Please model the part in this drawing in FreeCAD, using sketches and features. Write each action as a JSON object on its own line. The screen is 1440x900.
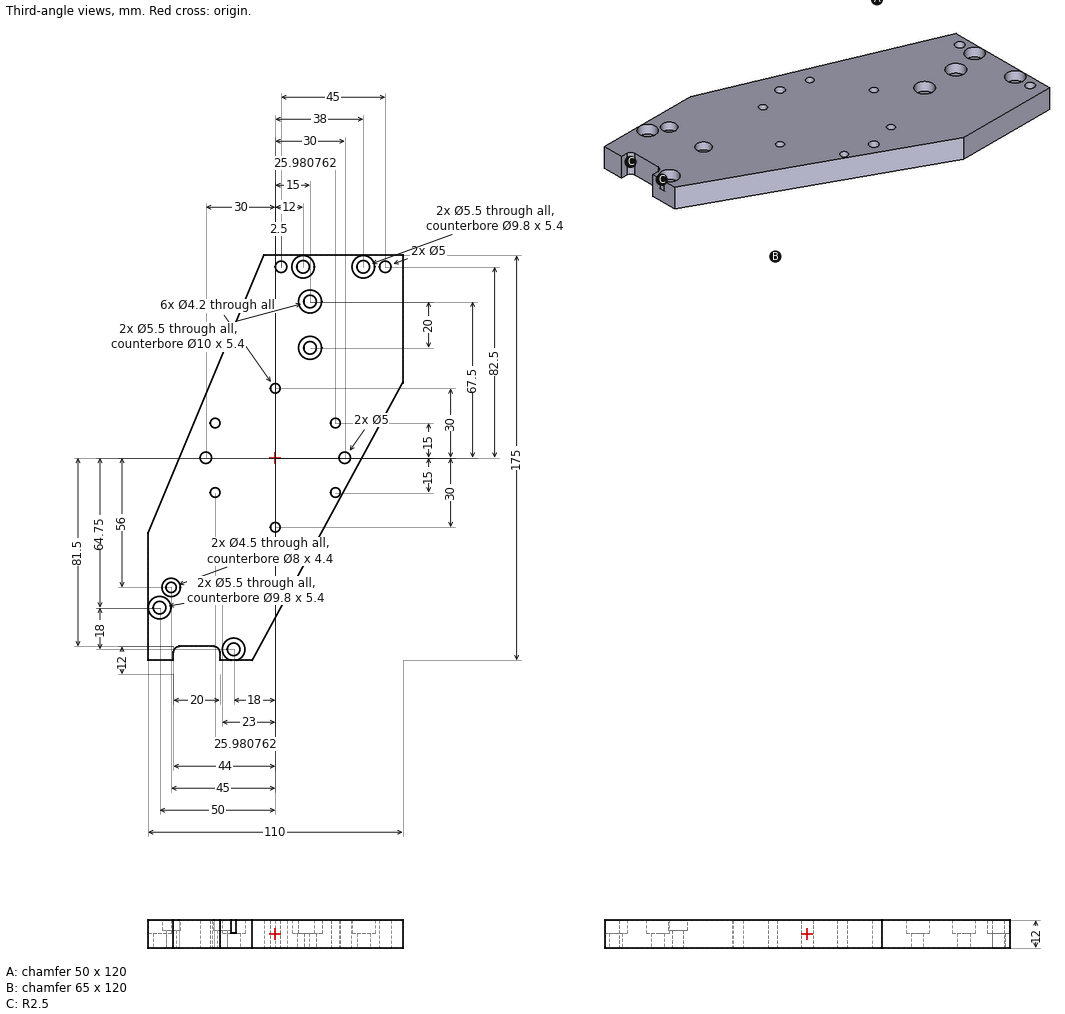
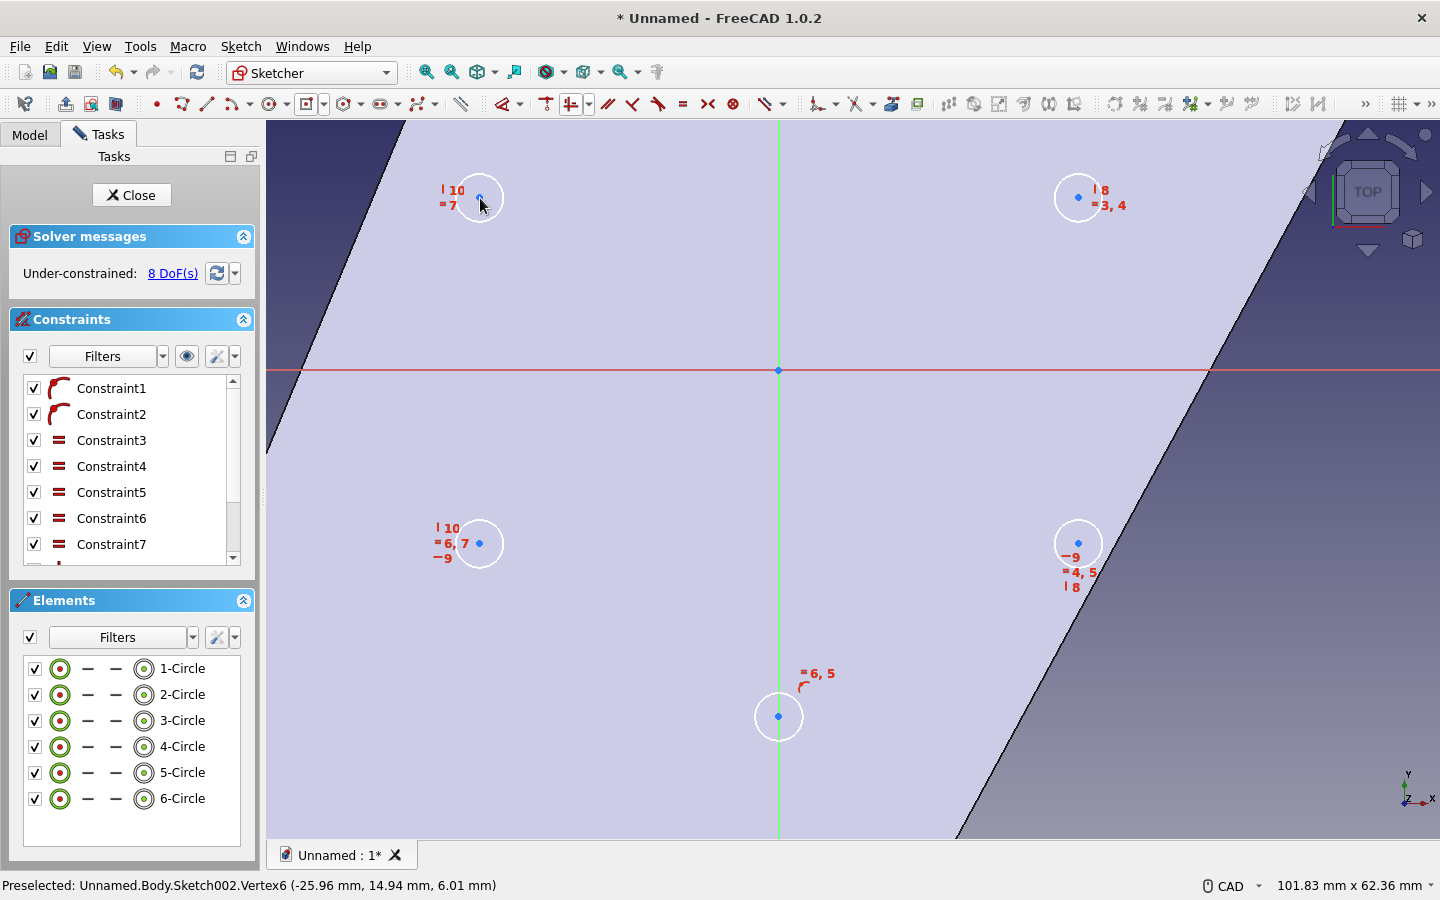
{"action": "left_click", "coordinate": [1079, 198]}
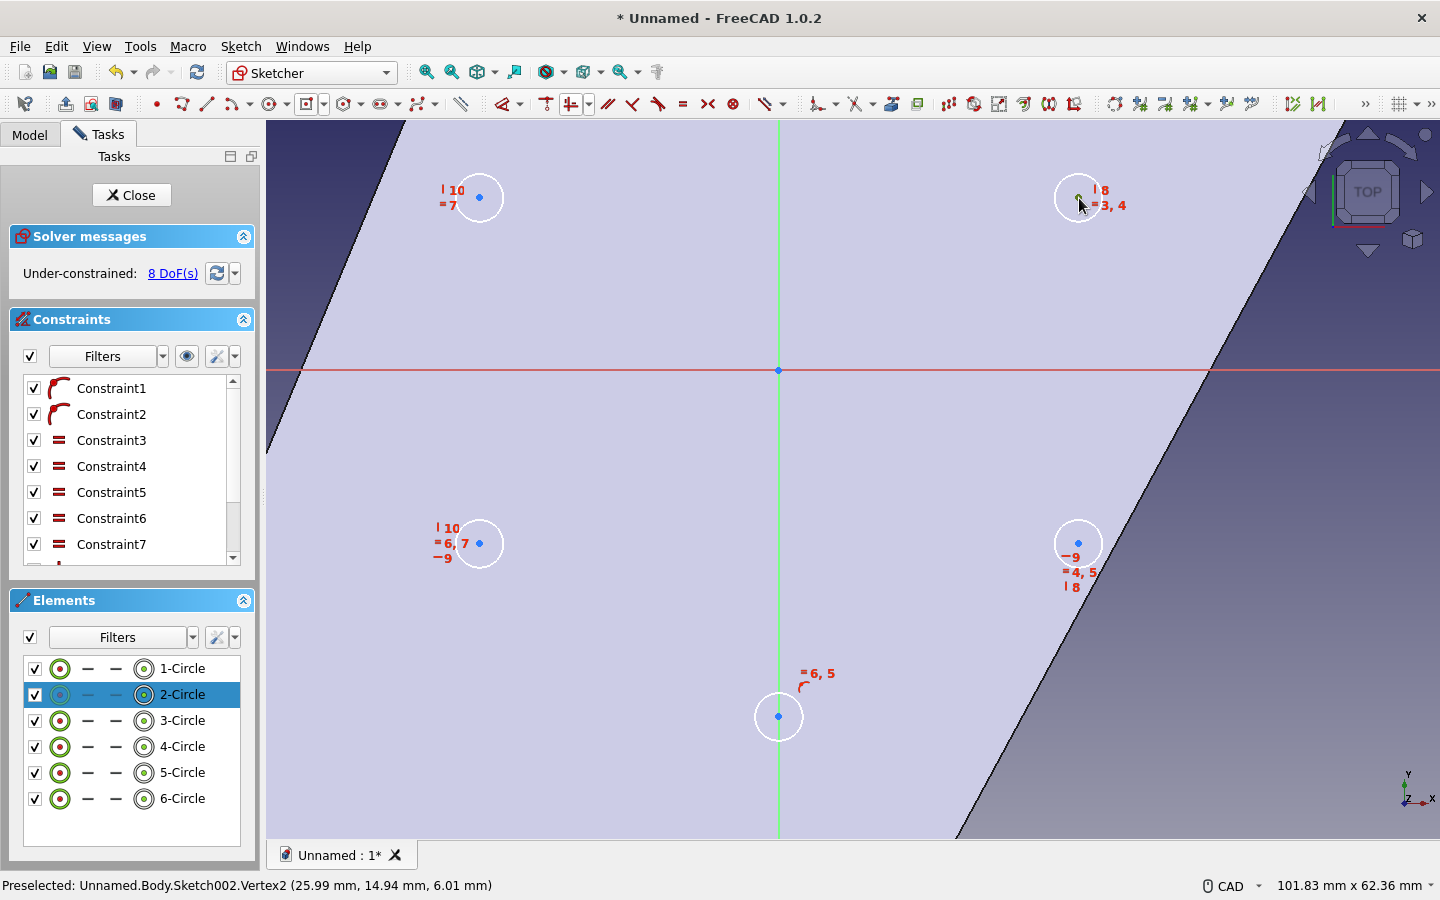
{"action": "left_click", "coordinate": [480, 198]}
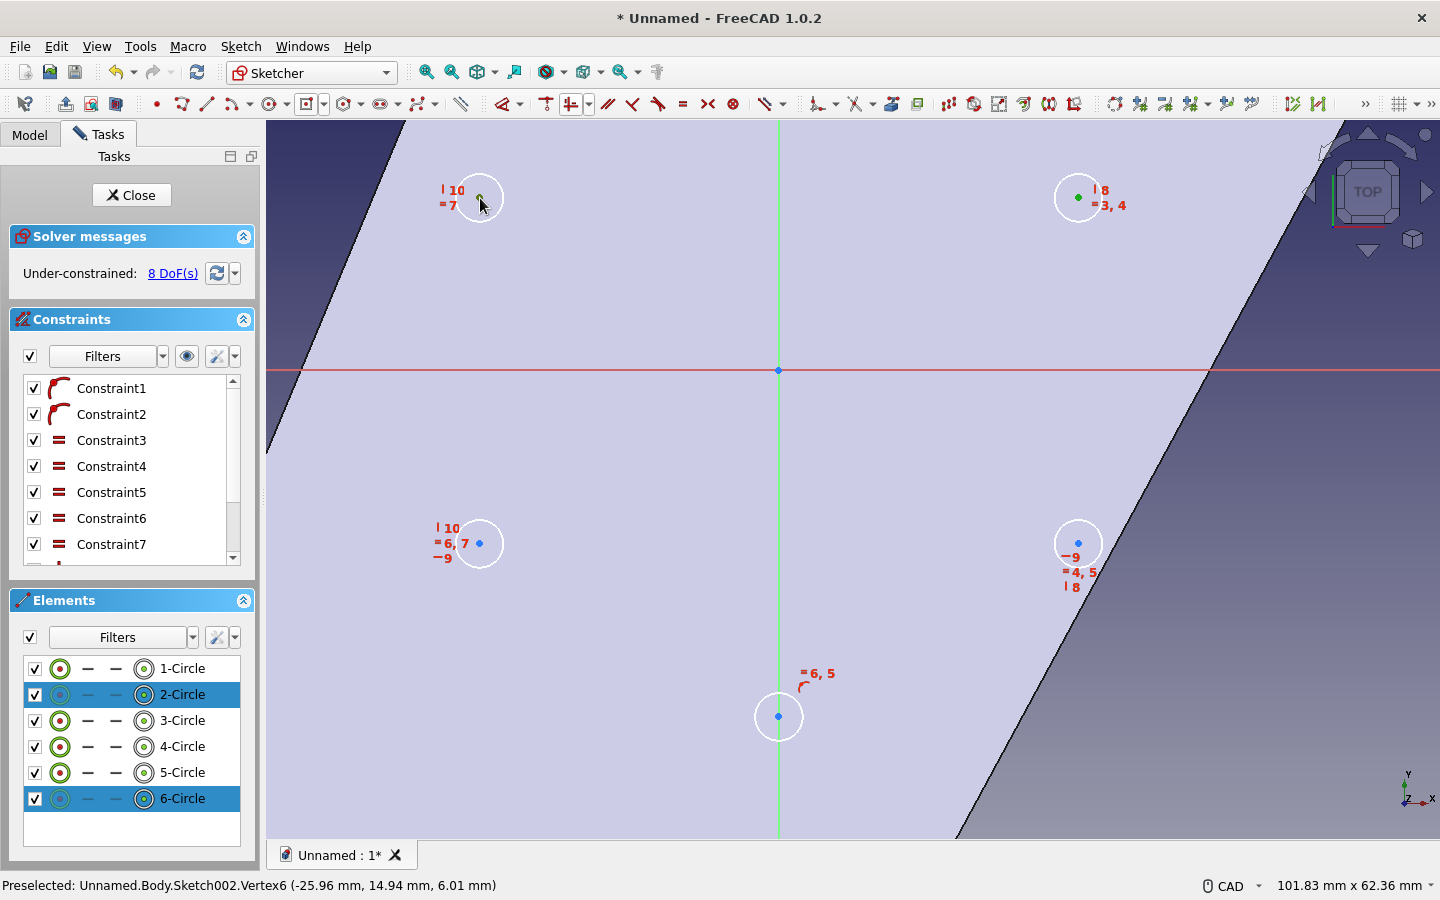
{"action": "key", "text": "h"}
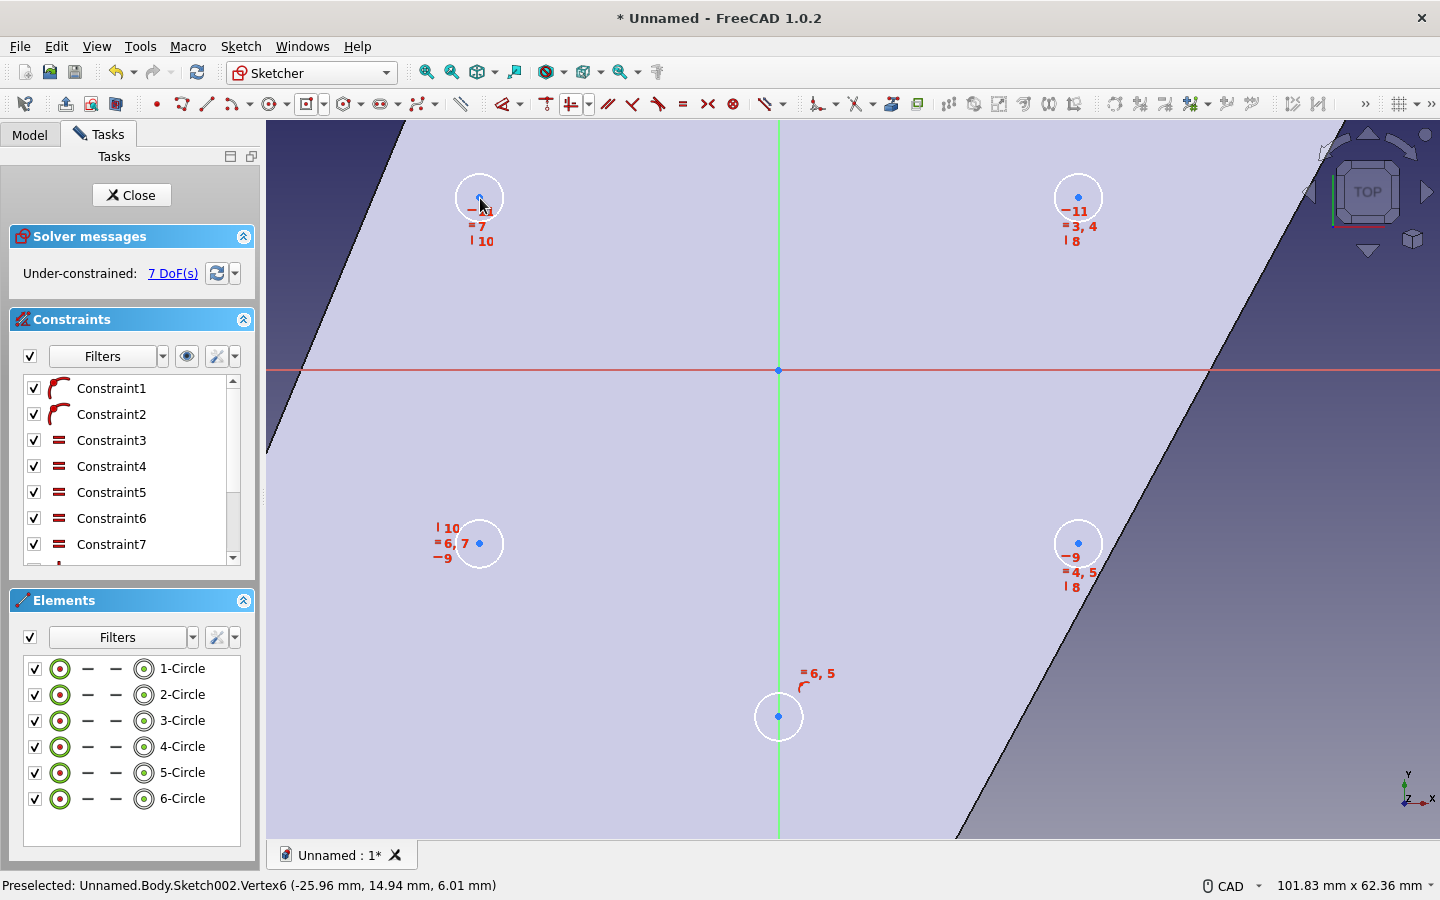
{"action": "scroll", "coordinate": [796, 702], "scroll_direction": "down", "scroll_amount": 2}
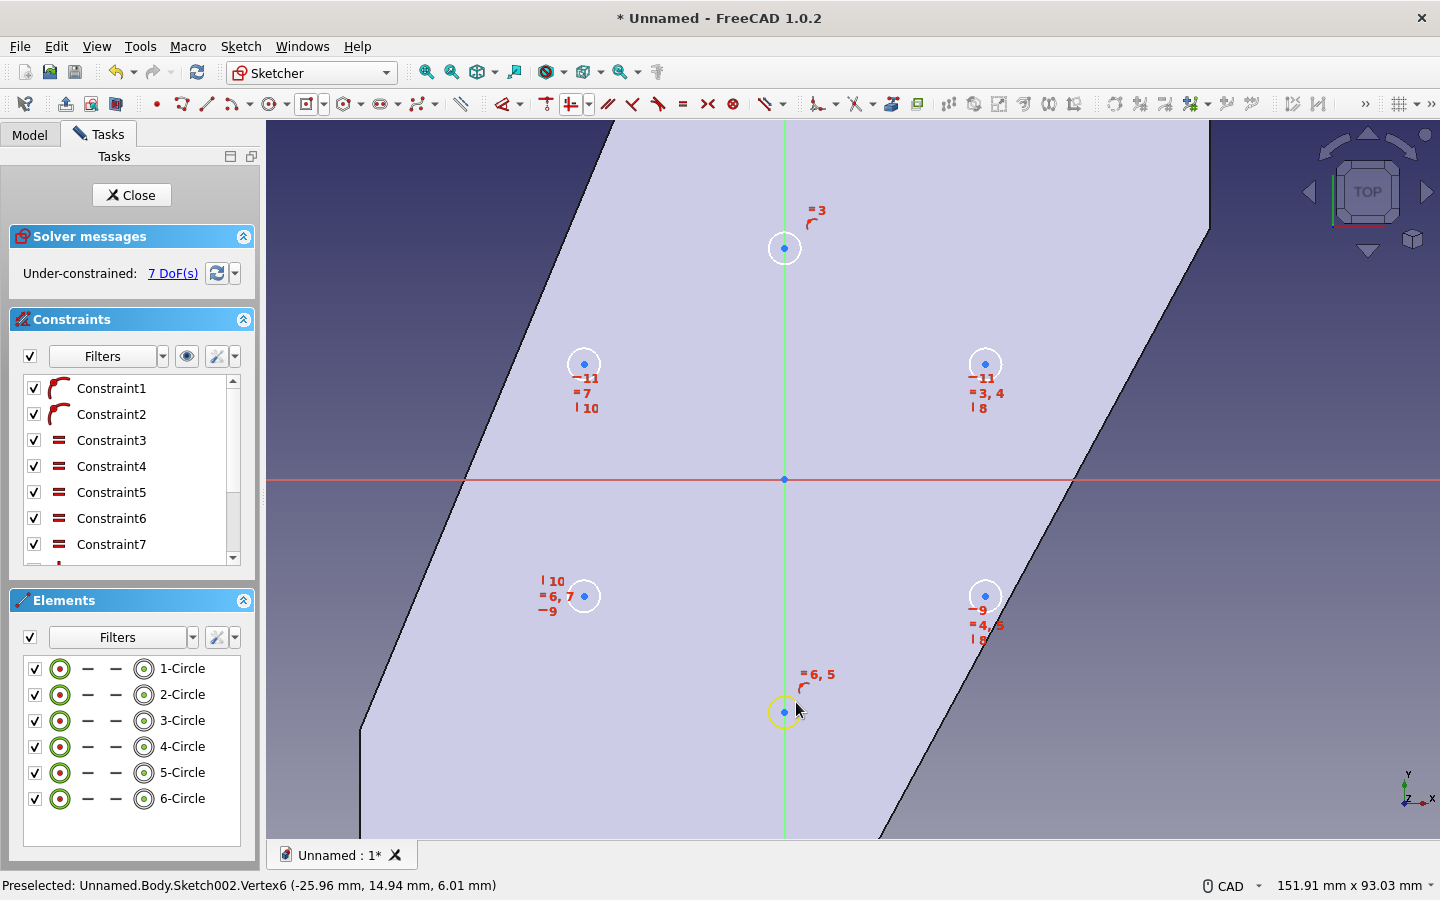
{"action": "scroll", "coordinate": [796, 237], "scroll_direction": "up", "scroll_amount": 2}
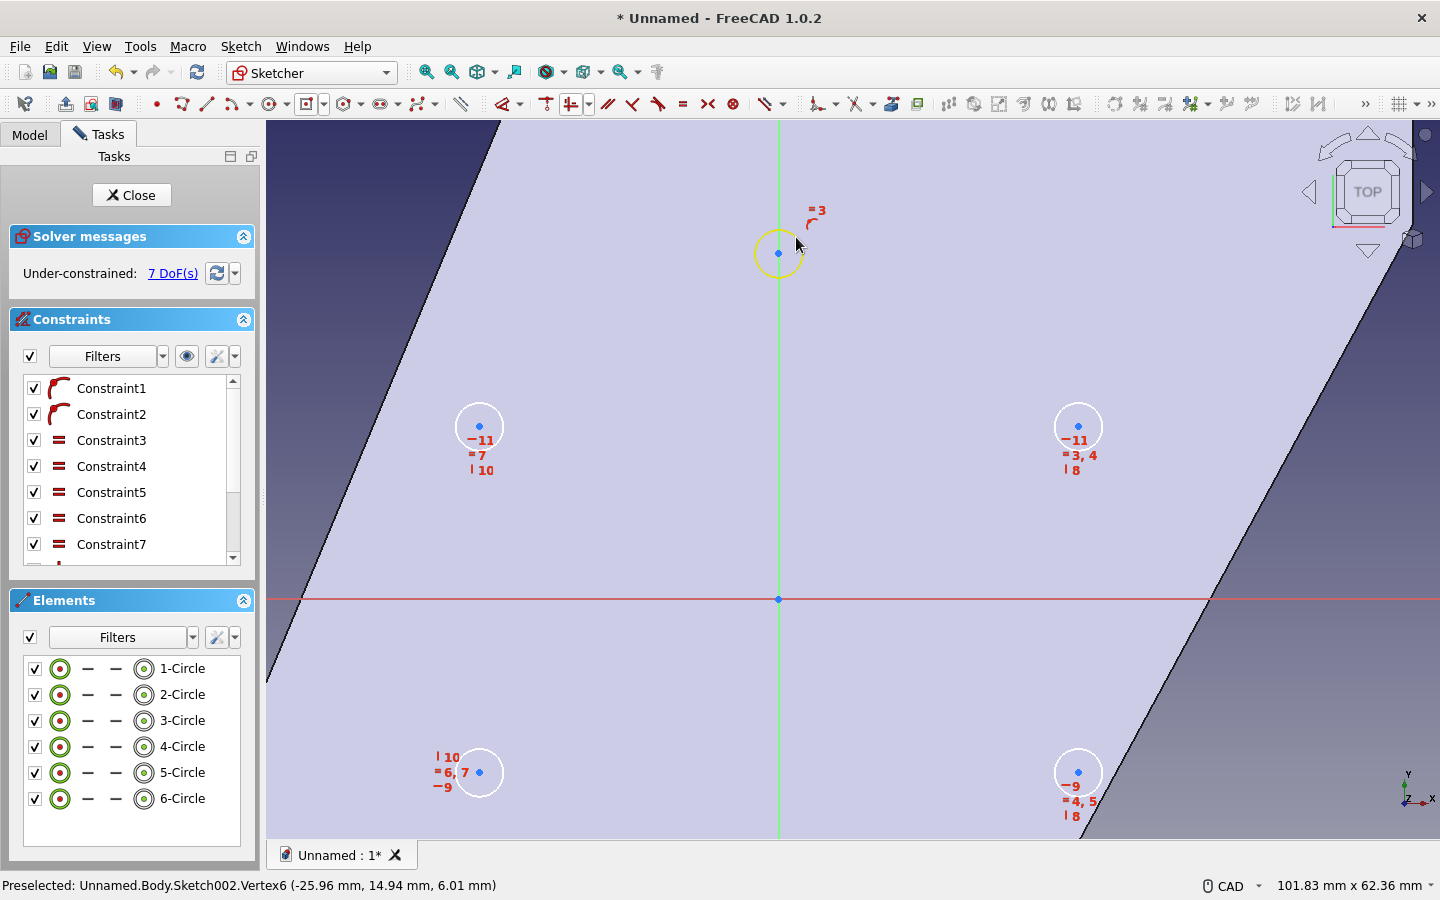
{"action": "left_click", "coordinate": [796, 237]}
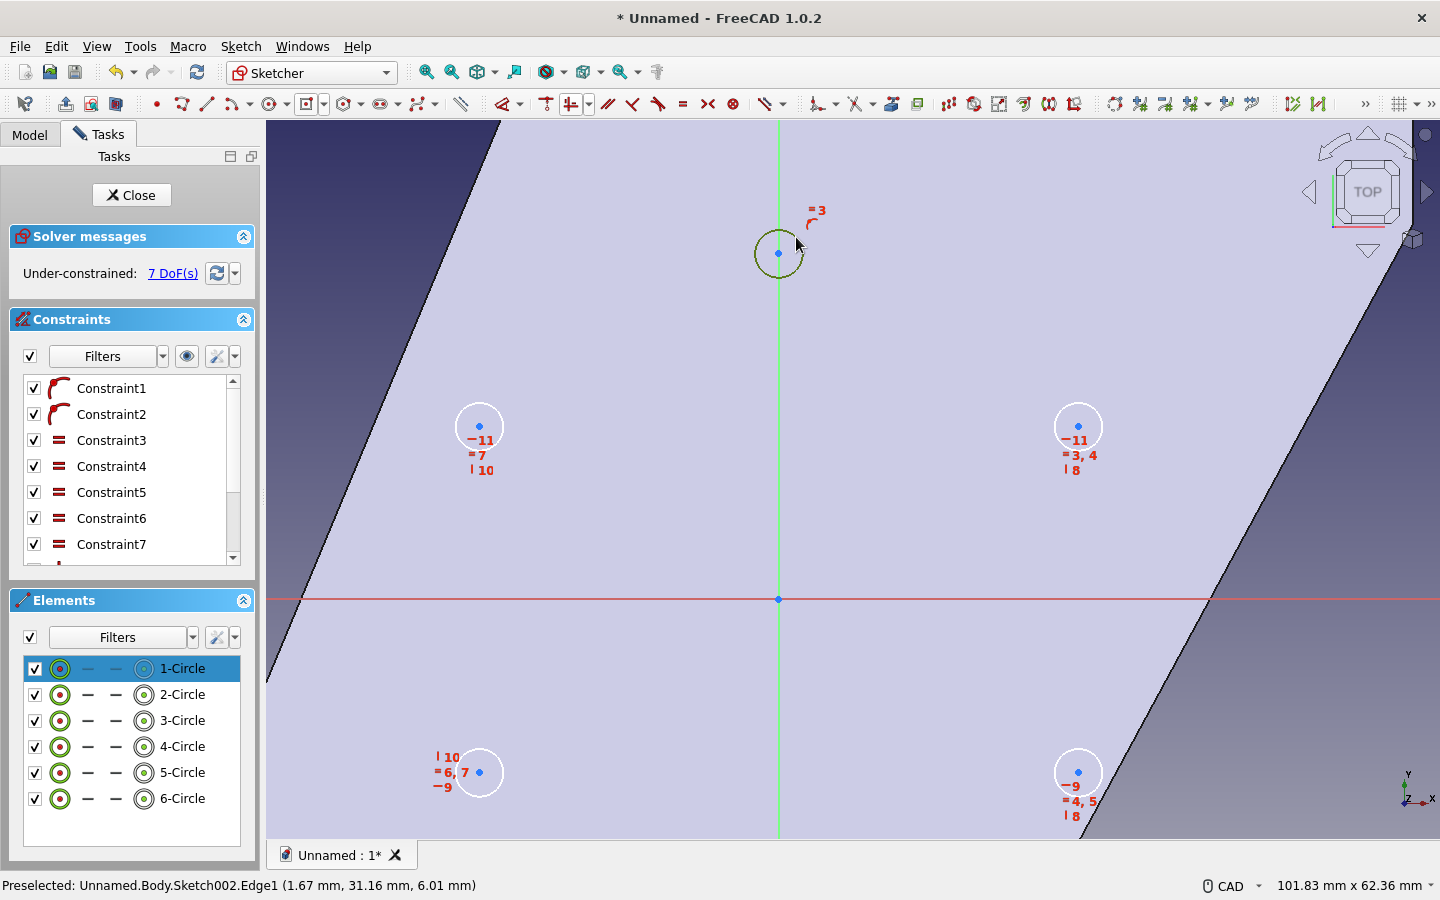
{"action": "key", "text": "k o"}